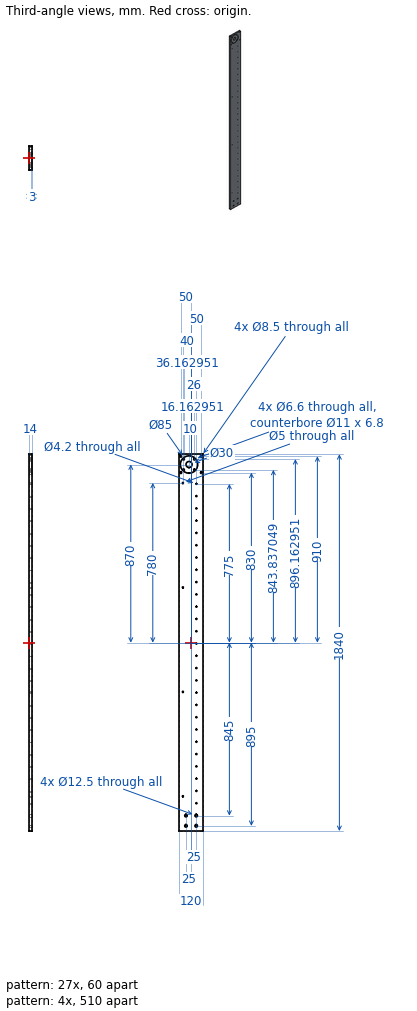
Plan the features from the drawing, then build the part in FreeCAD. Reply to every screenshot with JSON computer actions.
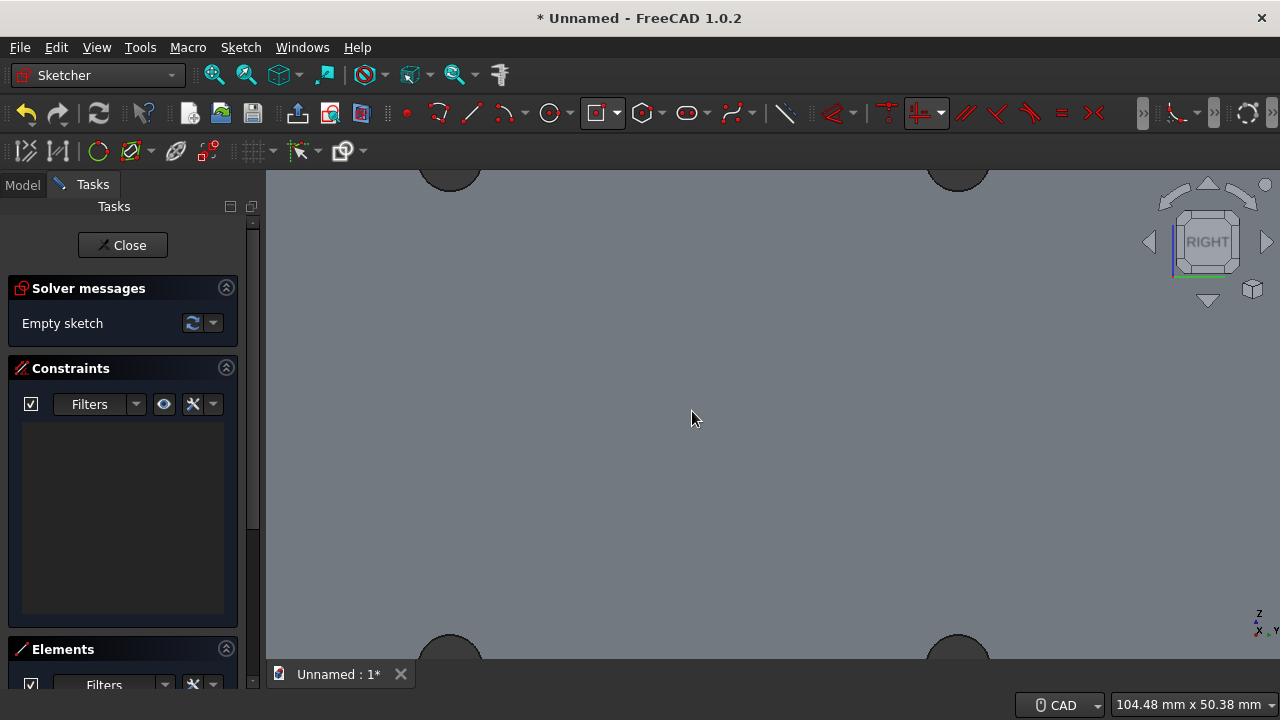
{"action": "left_click", "coordinate": [550, 114]}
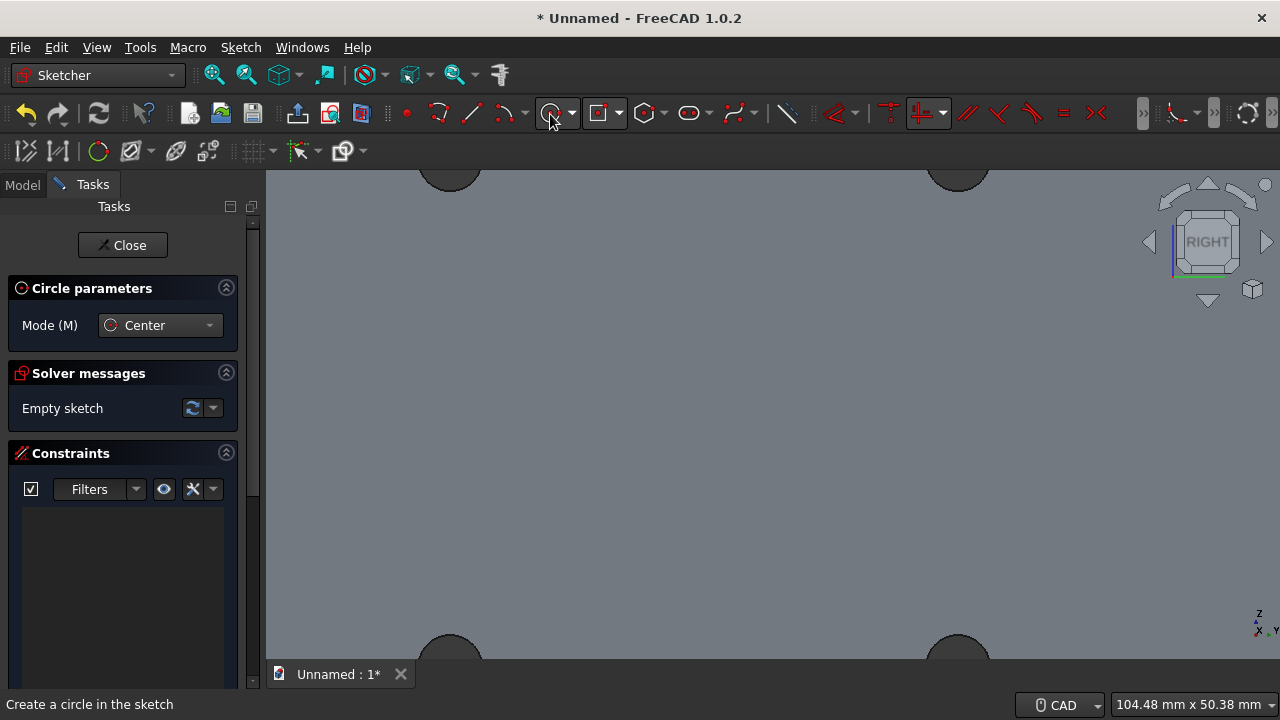
{"action": "left_click", "coordinate": [704, 413]}
{"action": "mouse_move", "coordinate": [601, 310]}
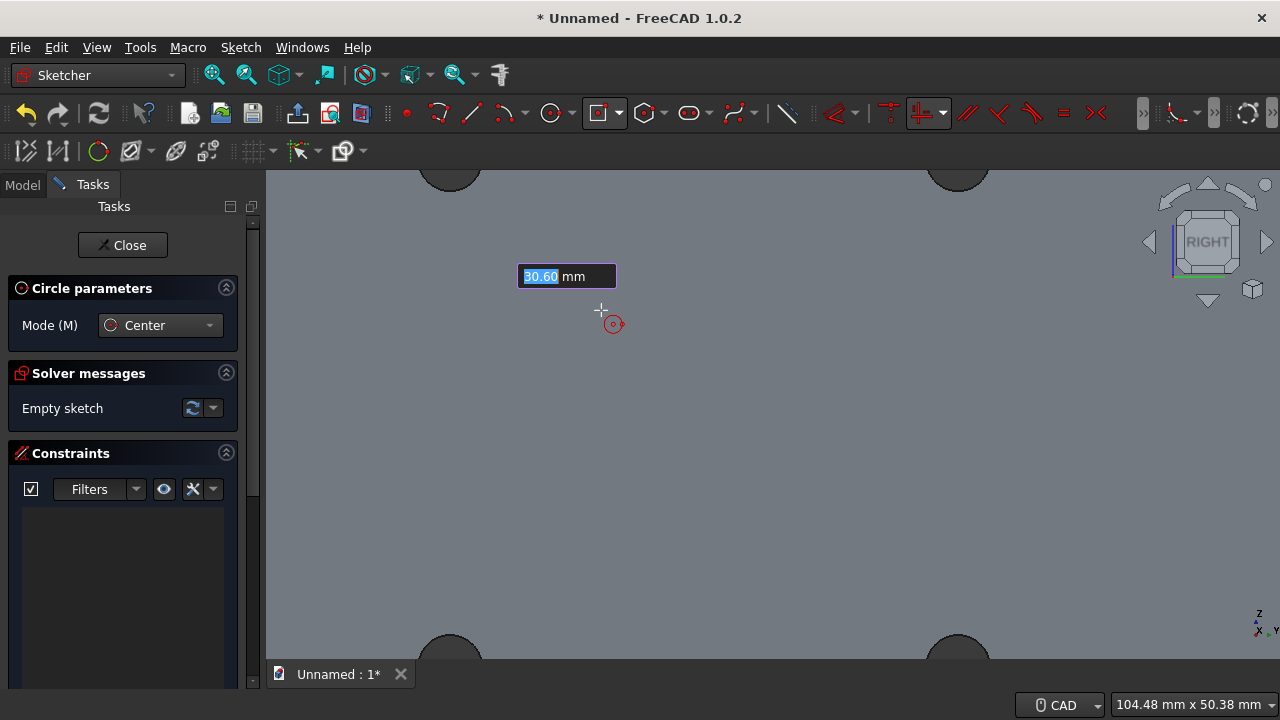
{"action": "type", "text": "30"}
{"action": "key", "text": "Return"}
{"action": "key", "text": "Escape"}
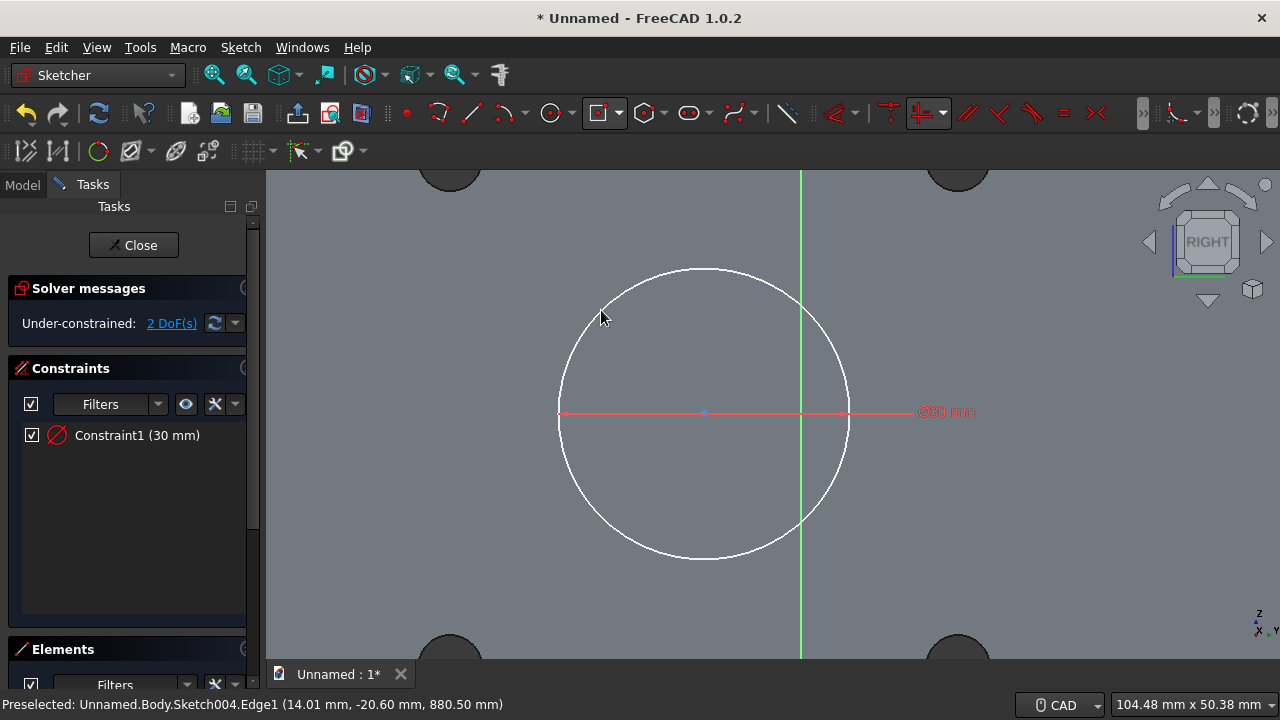
{"action": "left_click", "coordinate": [834, 114]}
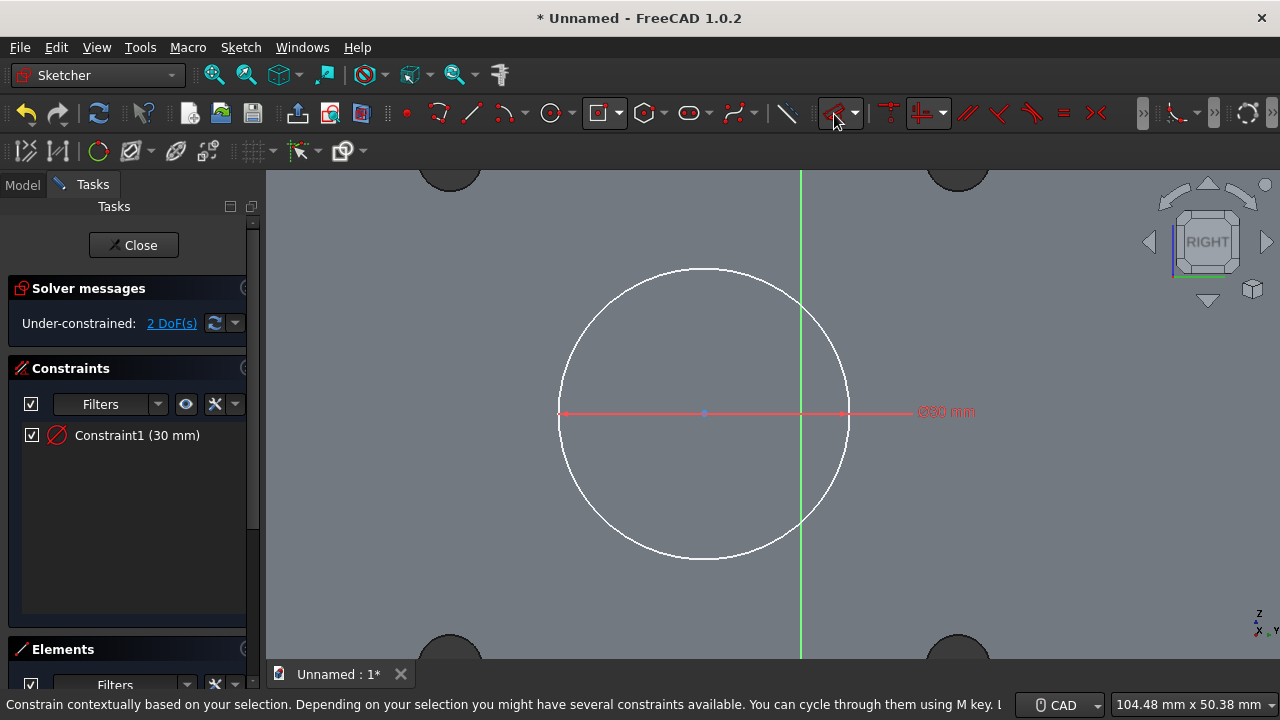
{"action": "left_click", "coordinate": [704, 414]}
{"action": "left_click", "coordinate": [753, 380]}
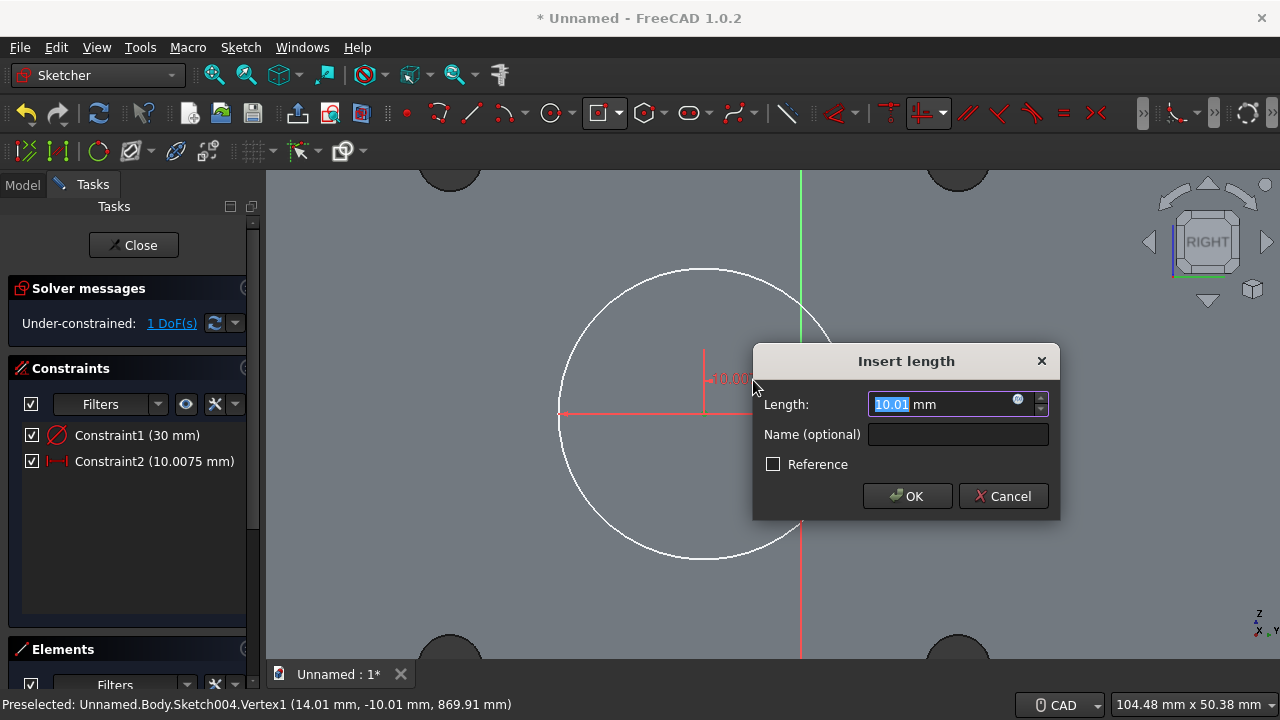
{"action": "type", "text": "10"}
{"action": "key", "text": "Return"}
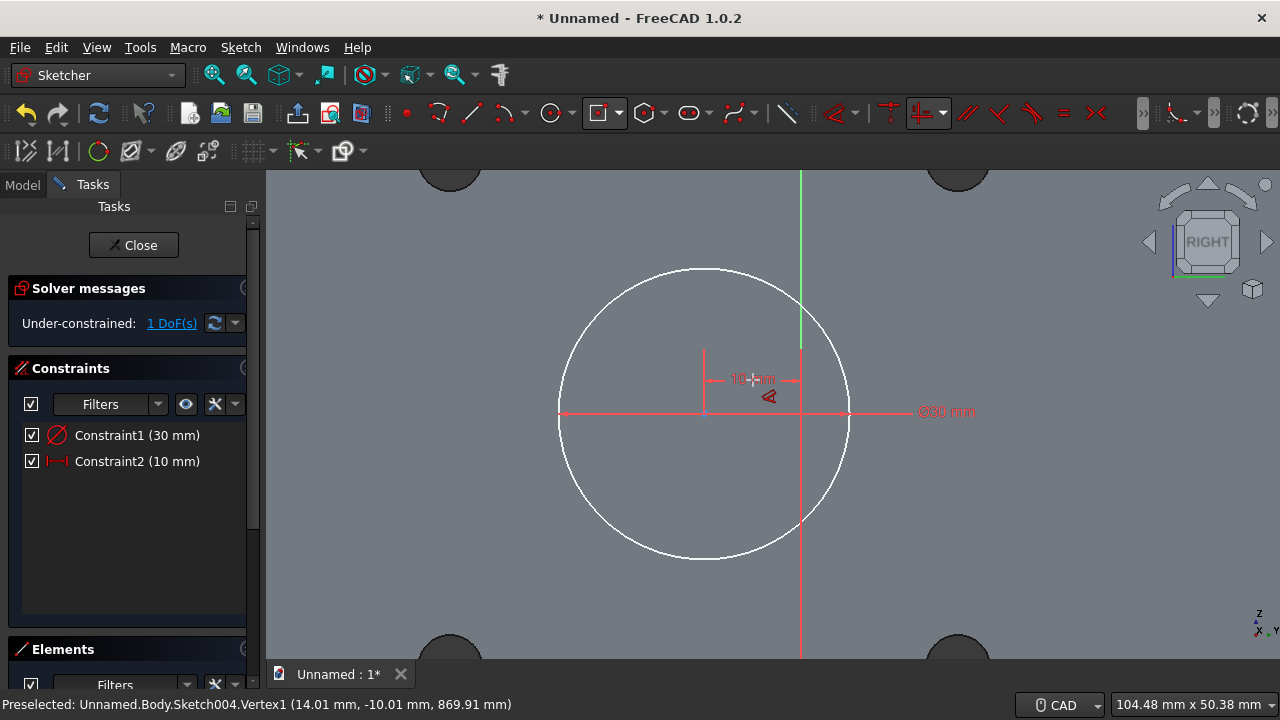
{"action": "left_click", "coordinate": [704, 414]}
{"action": "left_click", "coordinate": [835, 523]}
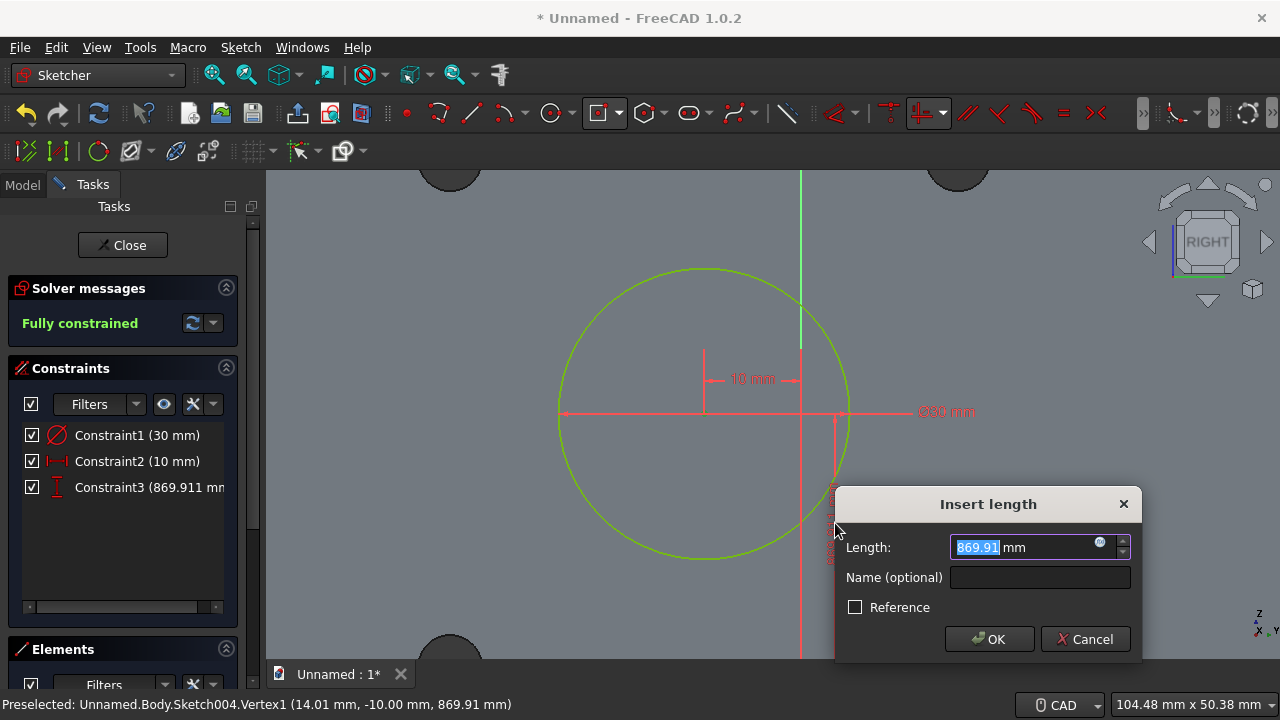
{"action": "type", "text": "870"}
{"action": "key", "text": "Return"}
{"action": "key", "text": "Escape"}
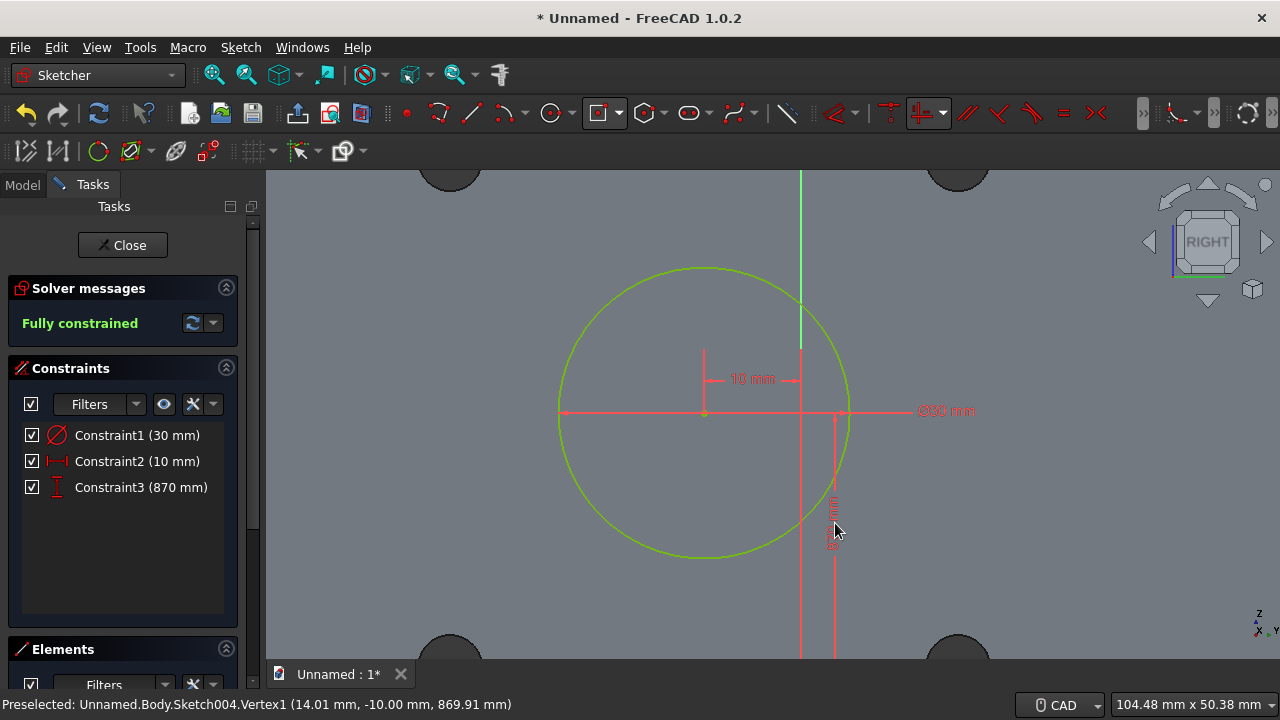
{"action": "left_click", "coordinate": [123, 245]}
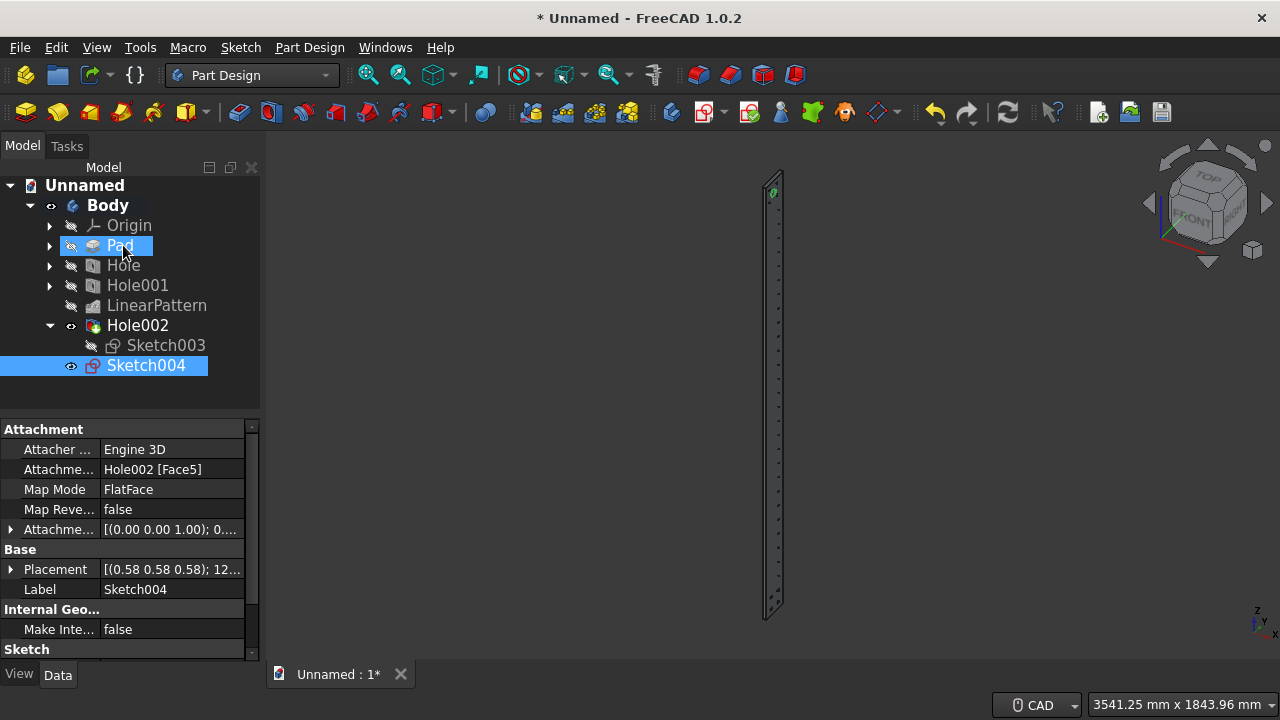
{"action": "left_click", "coordinate": [240, 112]}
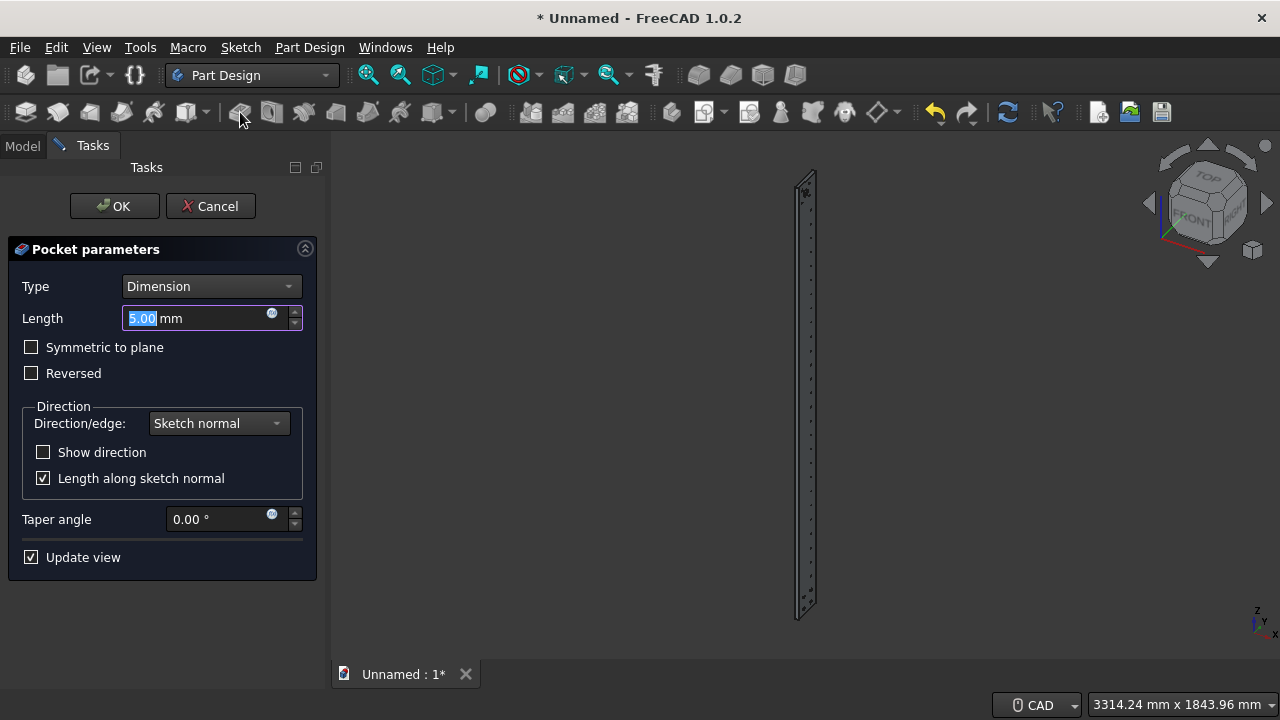
{"action": "left_click", "coordinate": [212, 286]}